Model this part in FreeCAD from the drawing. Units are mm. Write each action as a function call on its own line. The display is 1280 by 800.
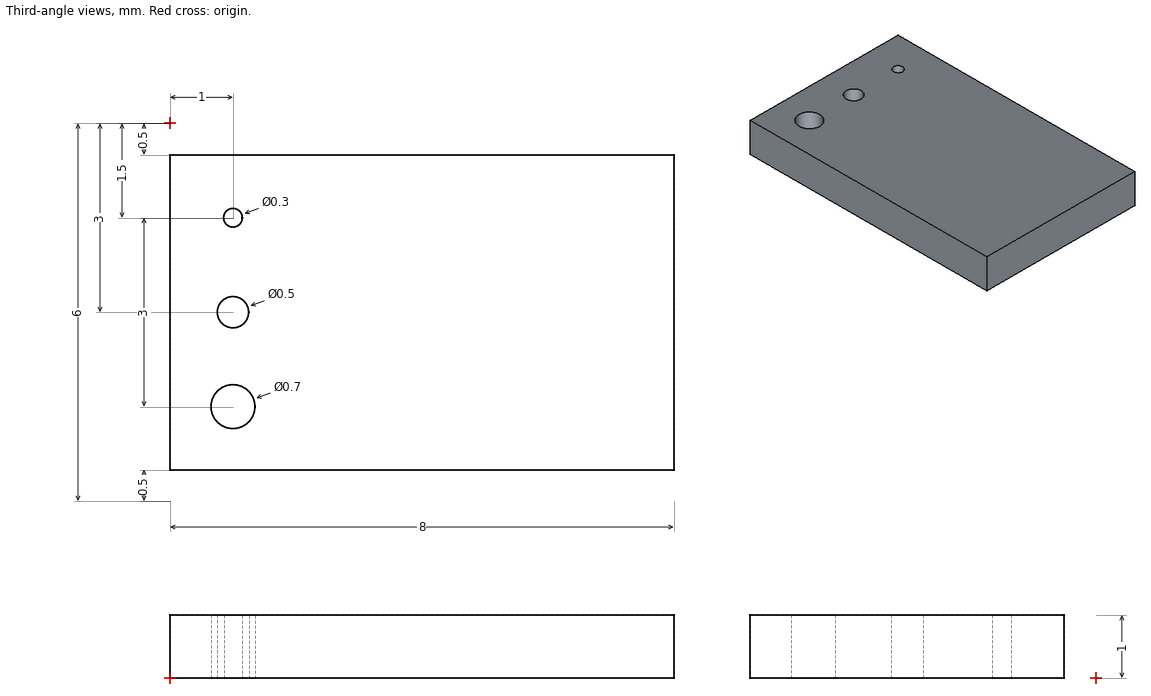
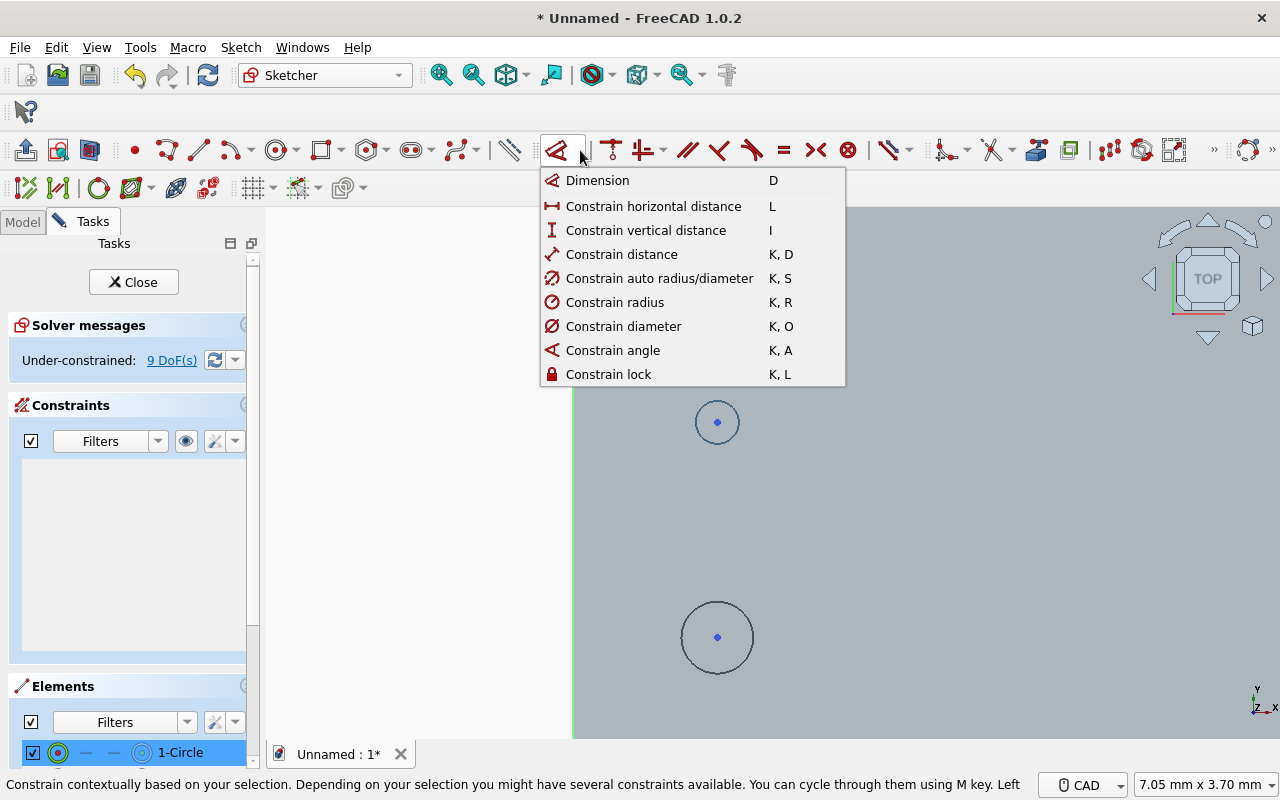
click(693, 326)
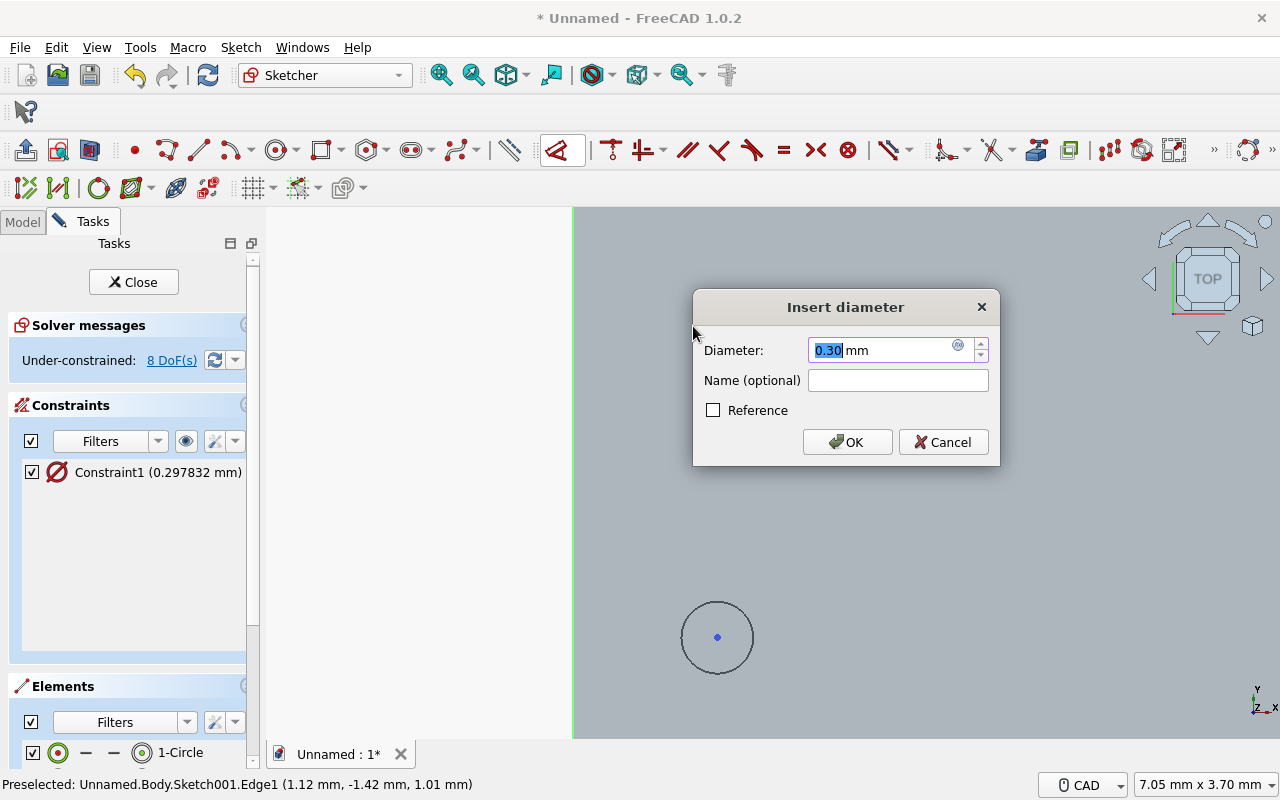
text(0.3)
key(Return)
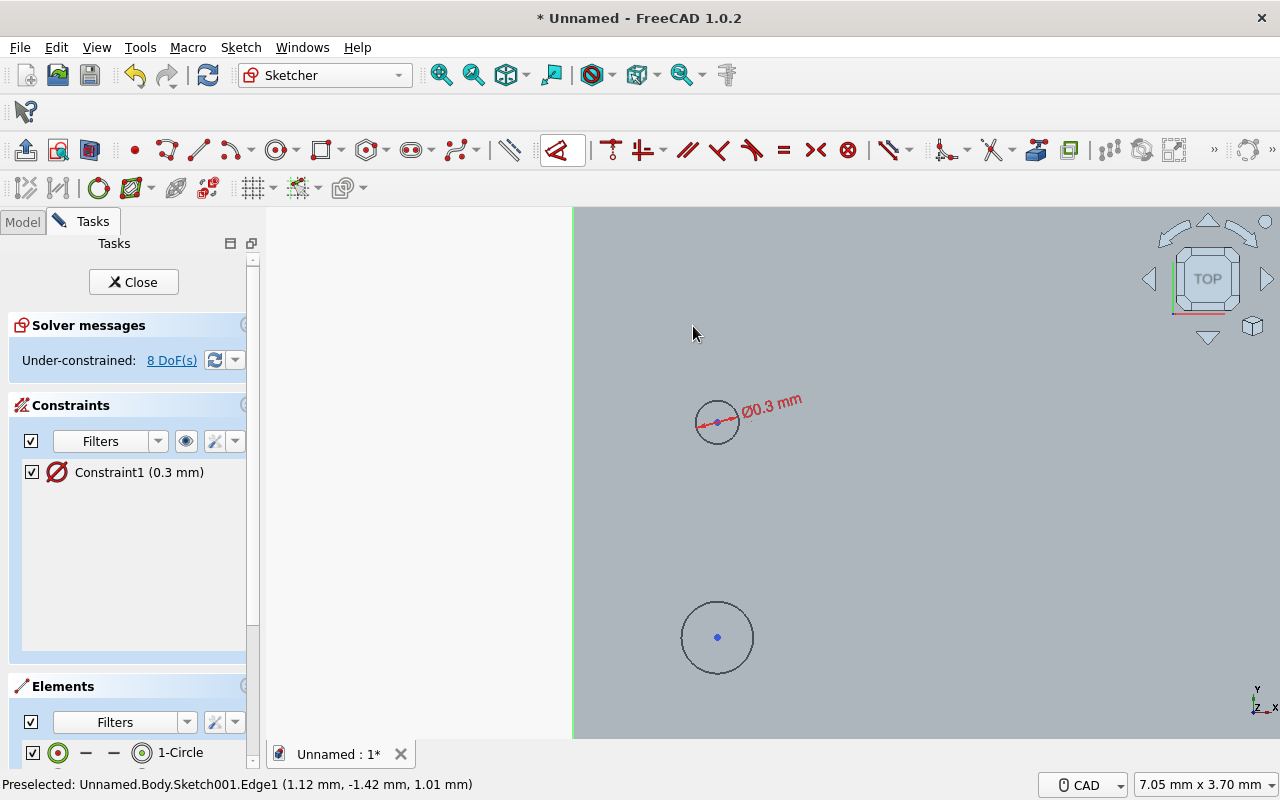
click(743, 612)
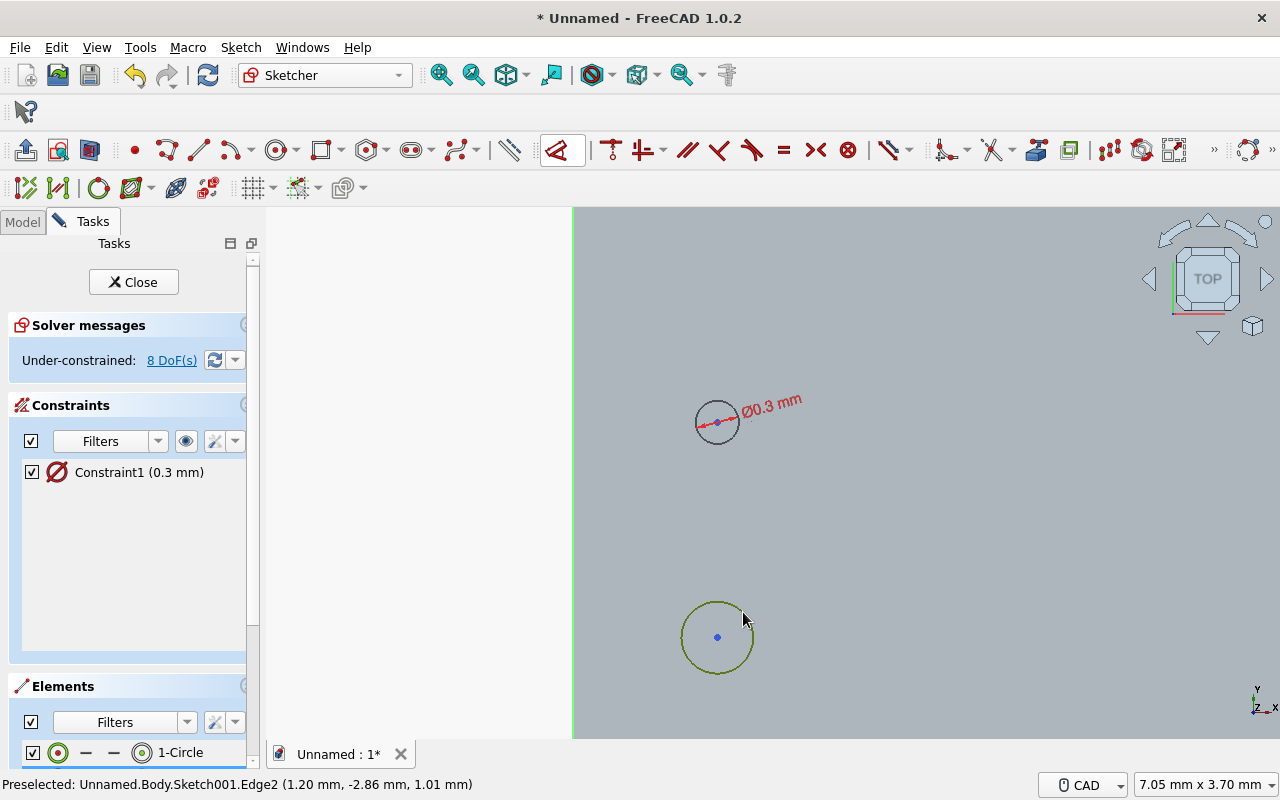
key(k)
key(o)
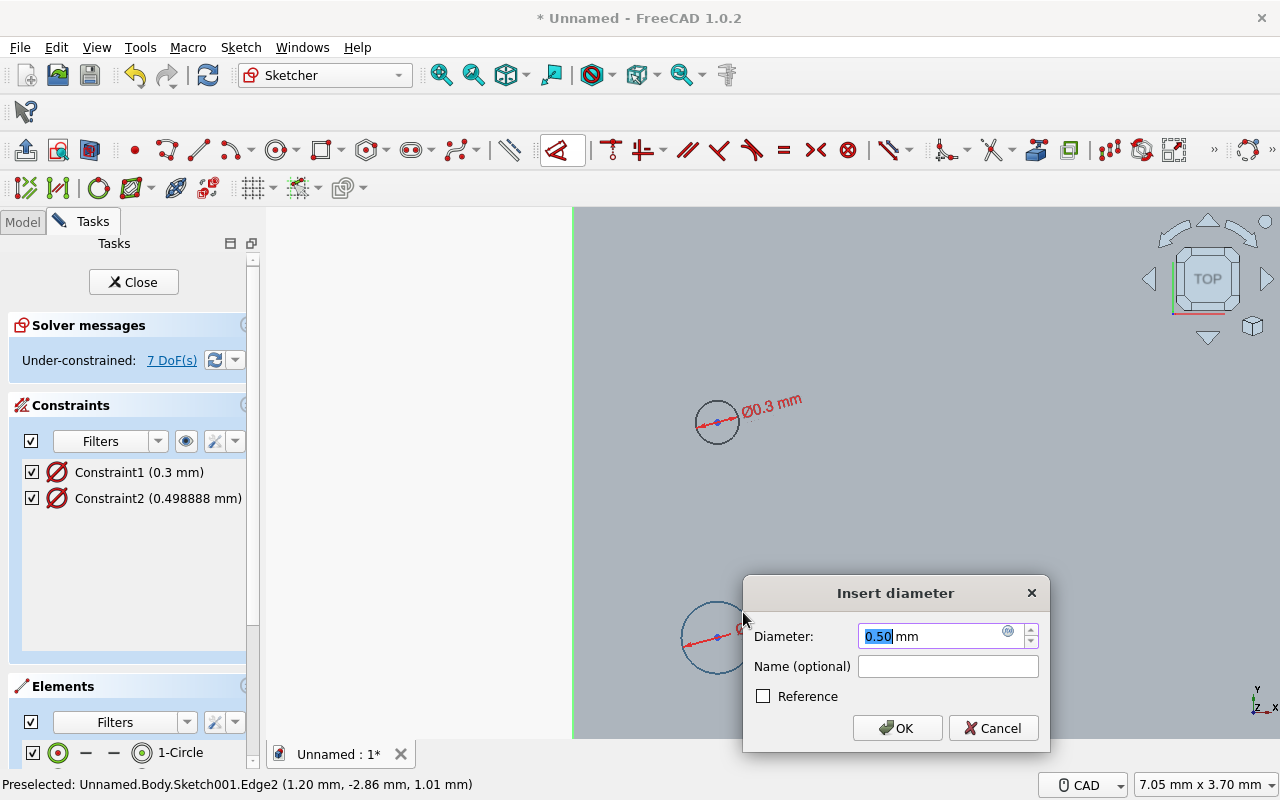
text(0.5)
key(Return)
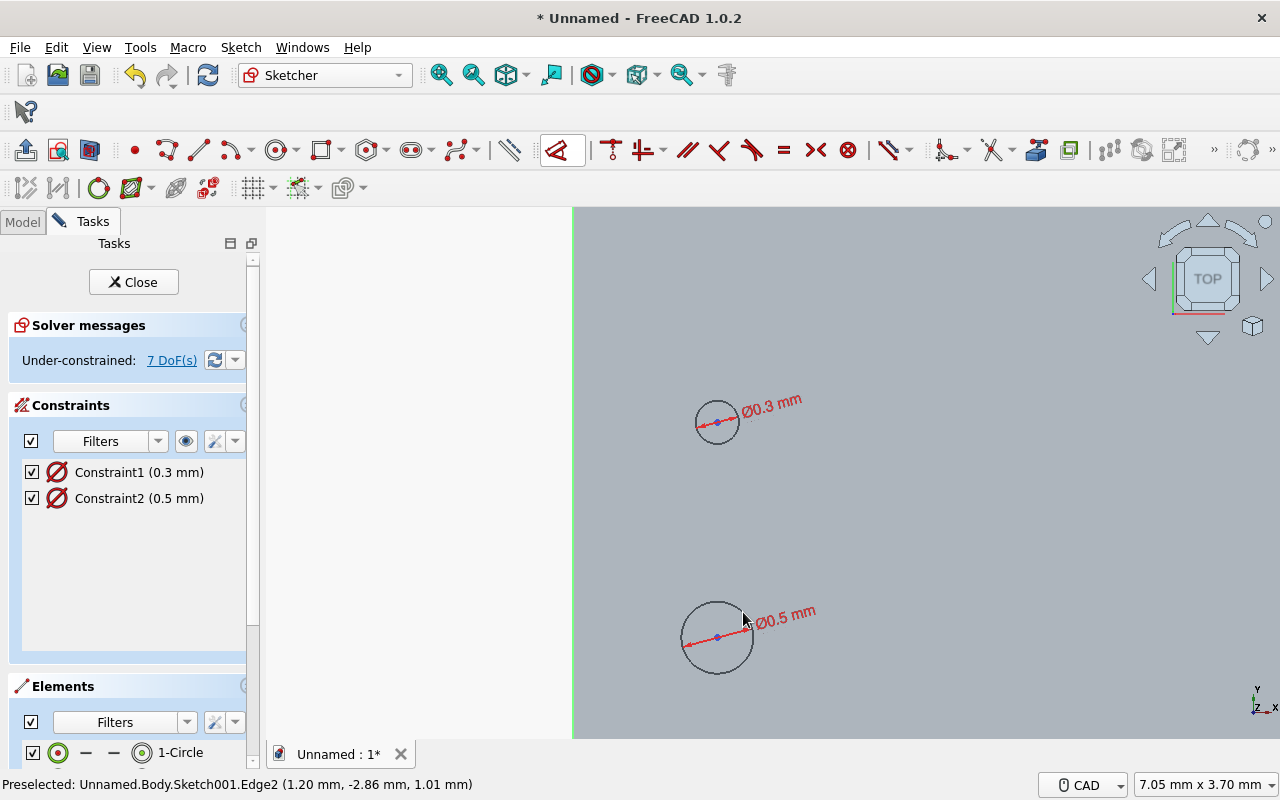
scroll(732, 406, down, 4)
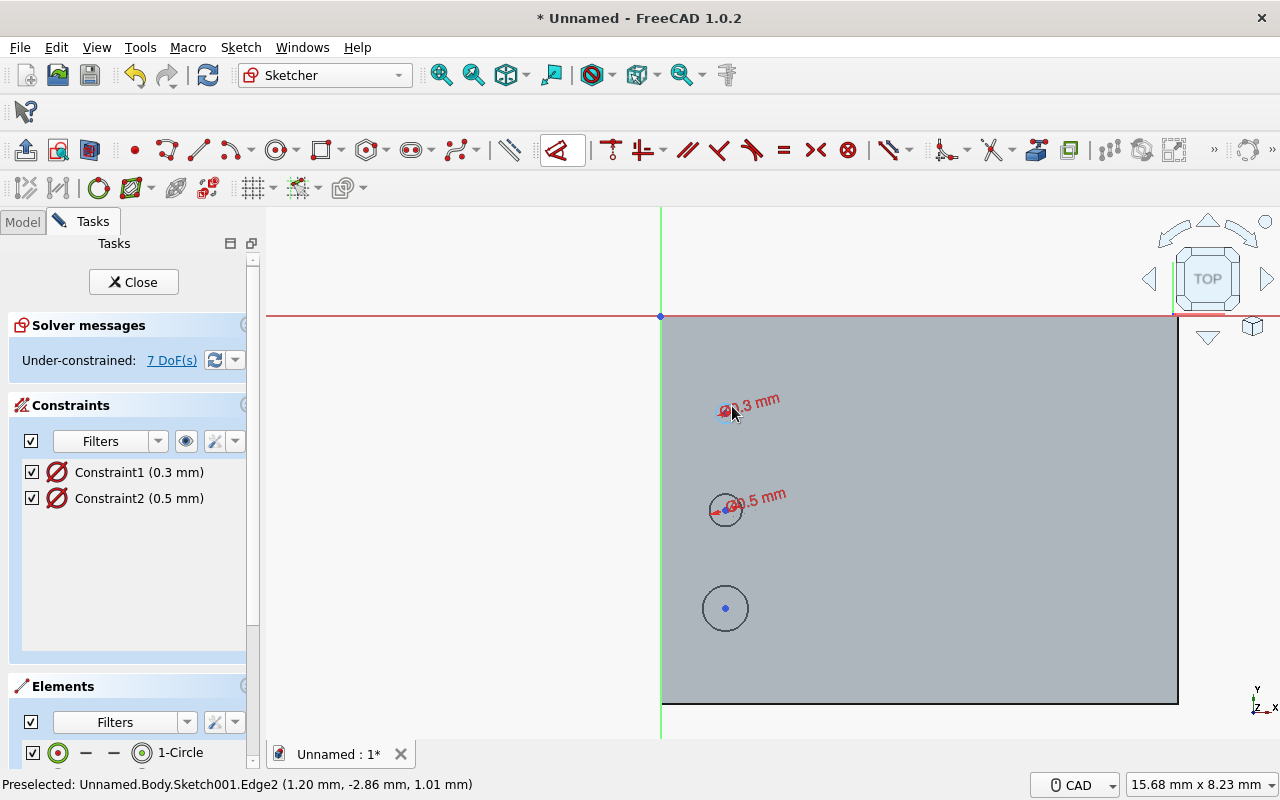
click(741, 592)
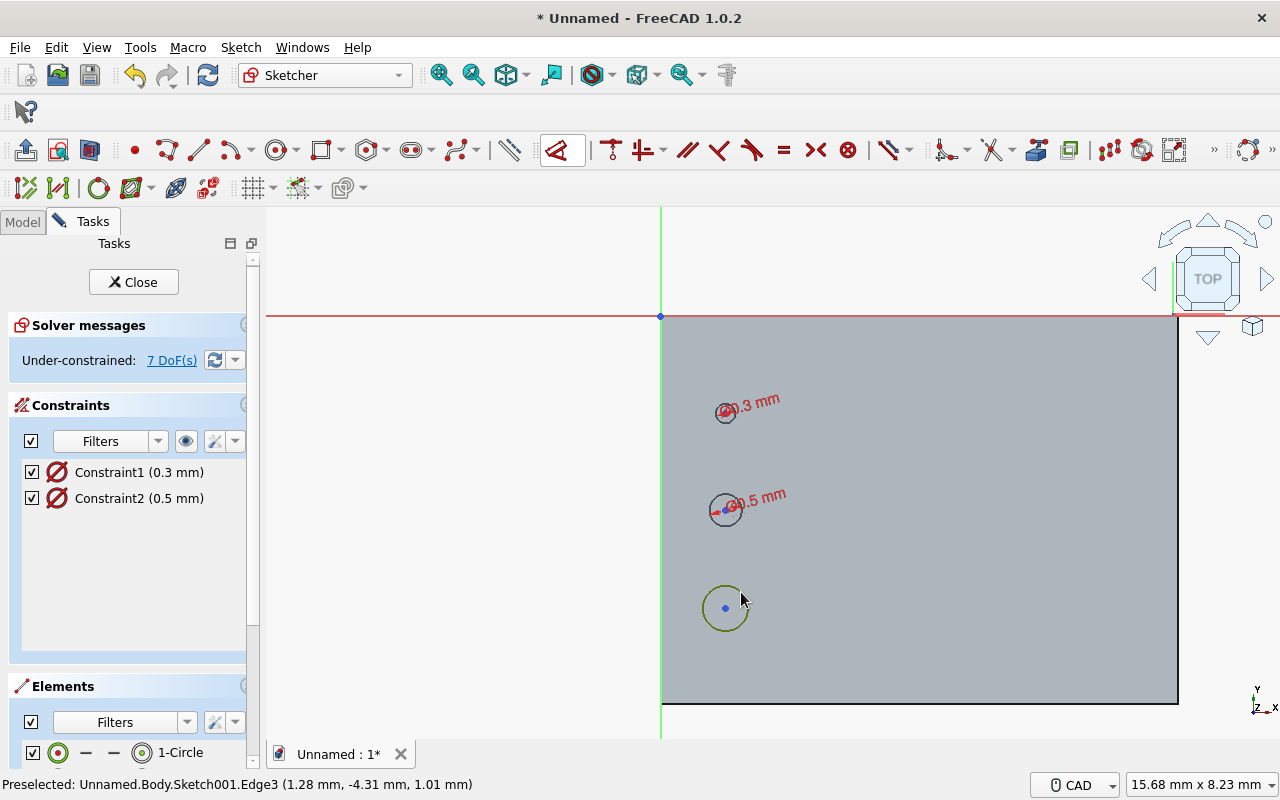
key(k)
key(o)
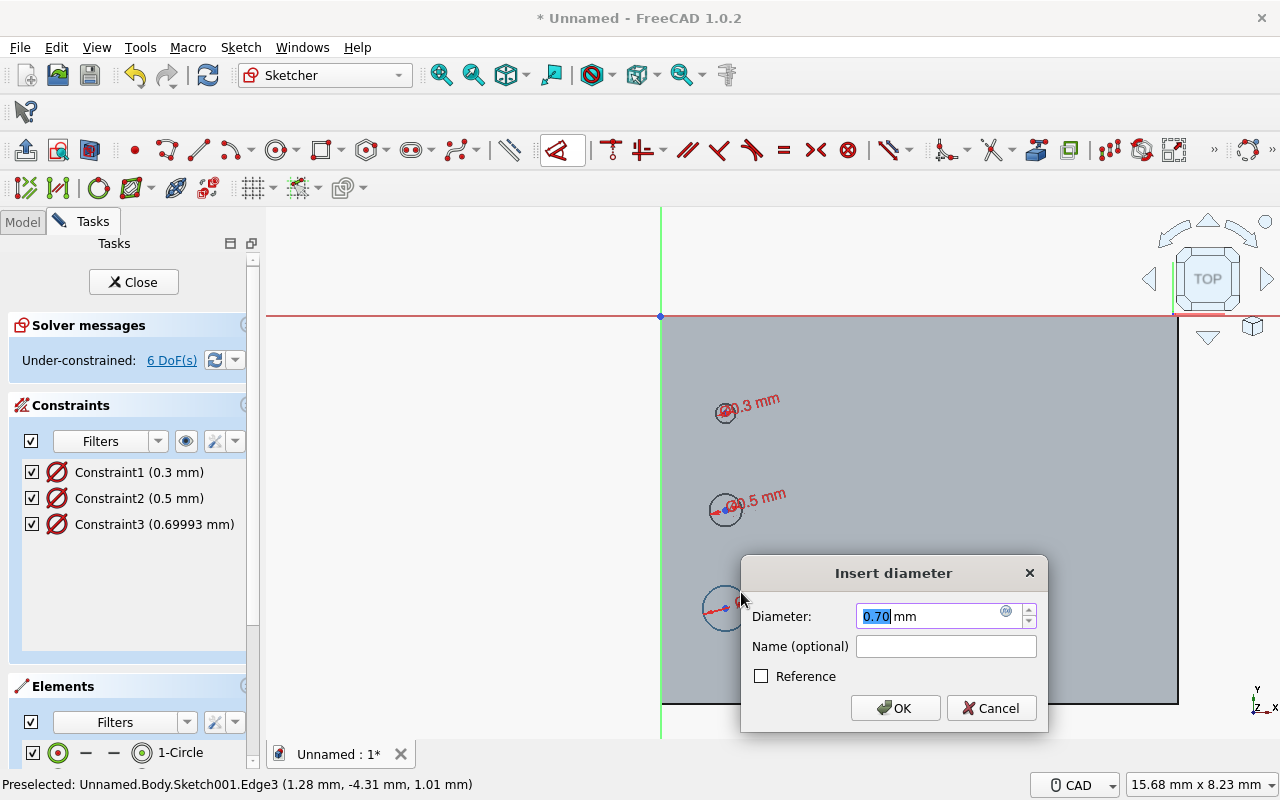
text(0.7)
key(Return)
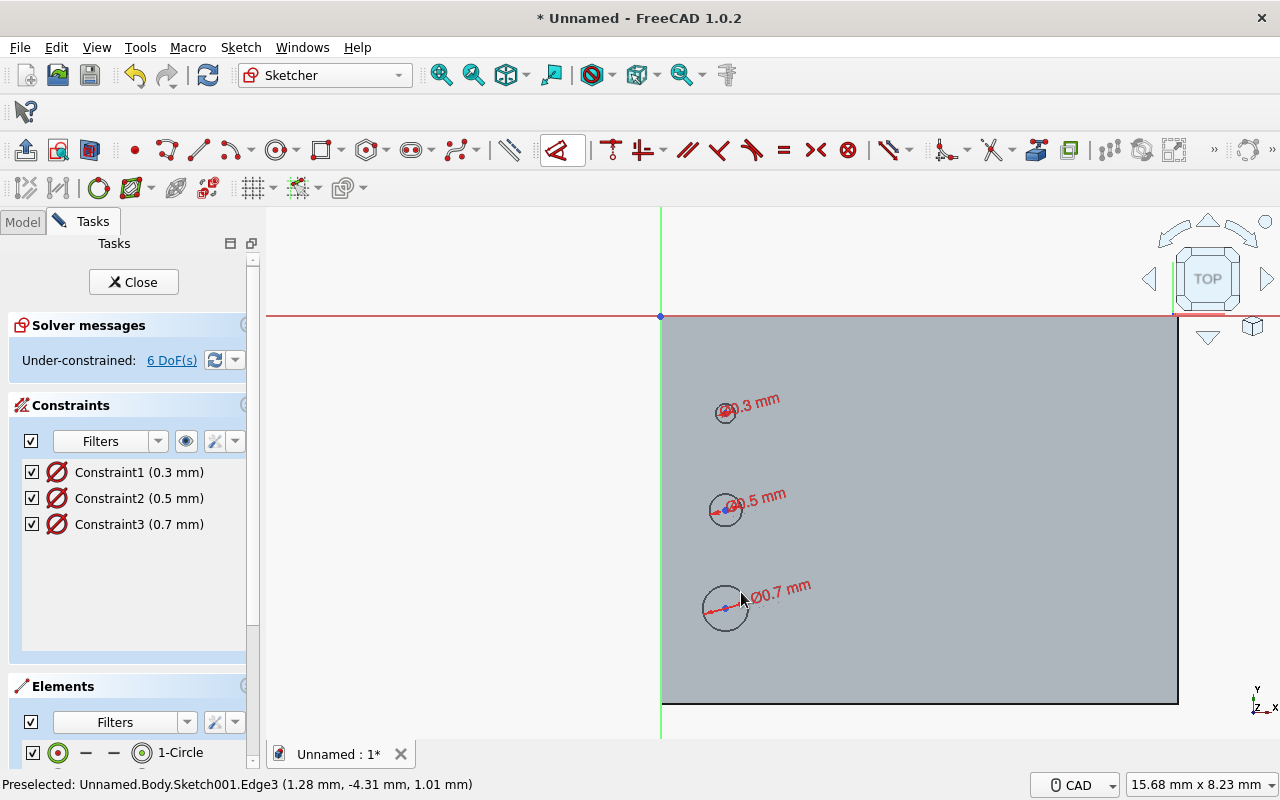
click(726, 414)